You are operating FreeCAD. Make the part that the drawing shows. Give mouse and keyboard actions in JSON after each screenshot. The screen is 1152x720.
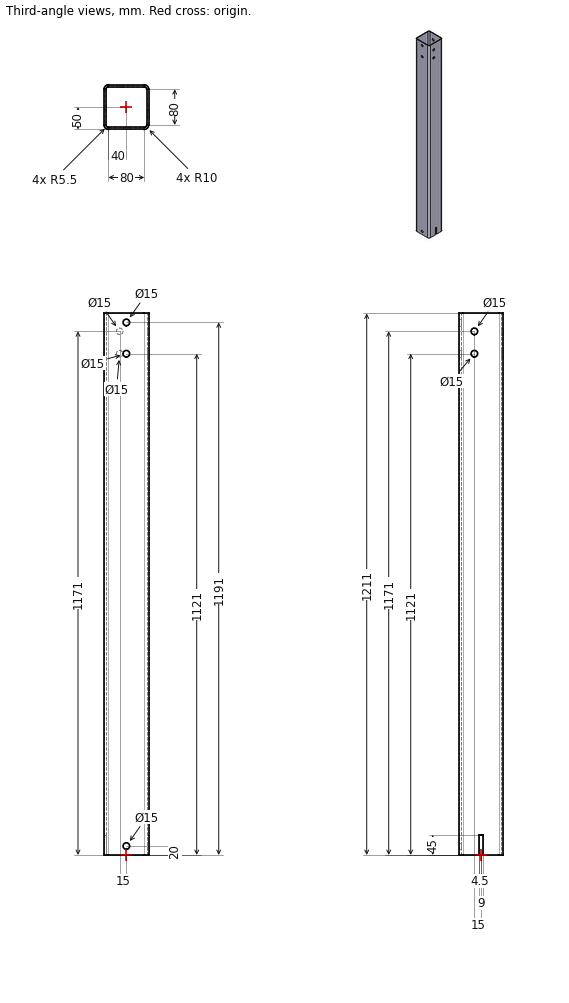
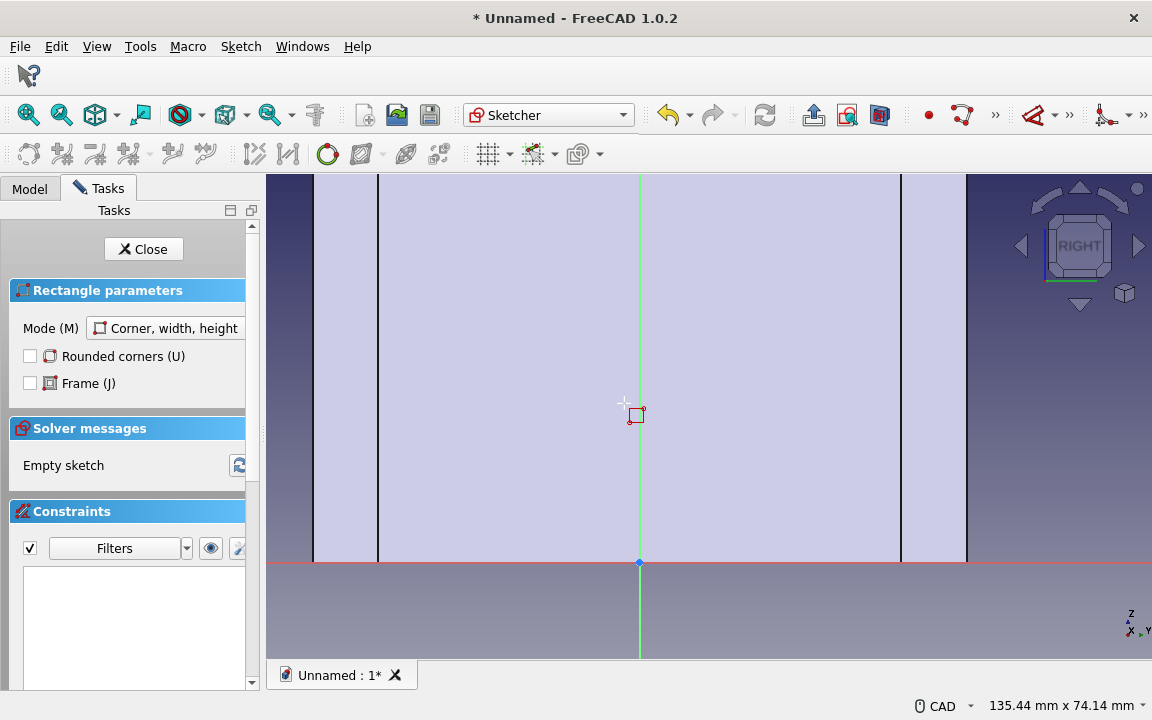
{"action": "left_click", "coordinate": [610, 268]}
{"action": "left_click", "coordinate": [669, 563]}
{"action": "key", "text": "Escape"}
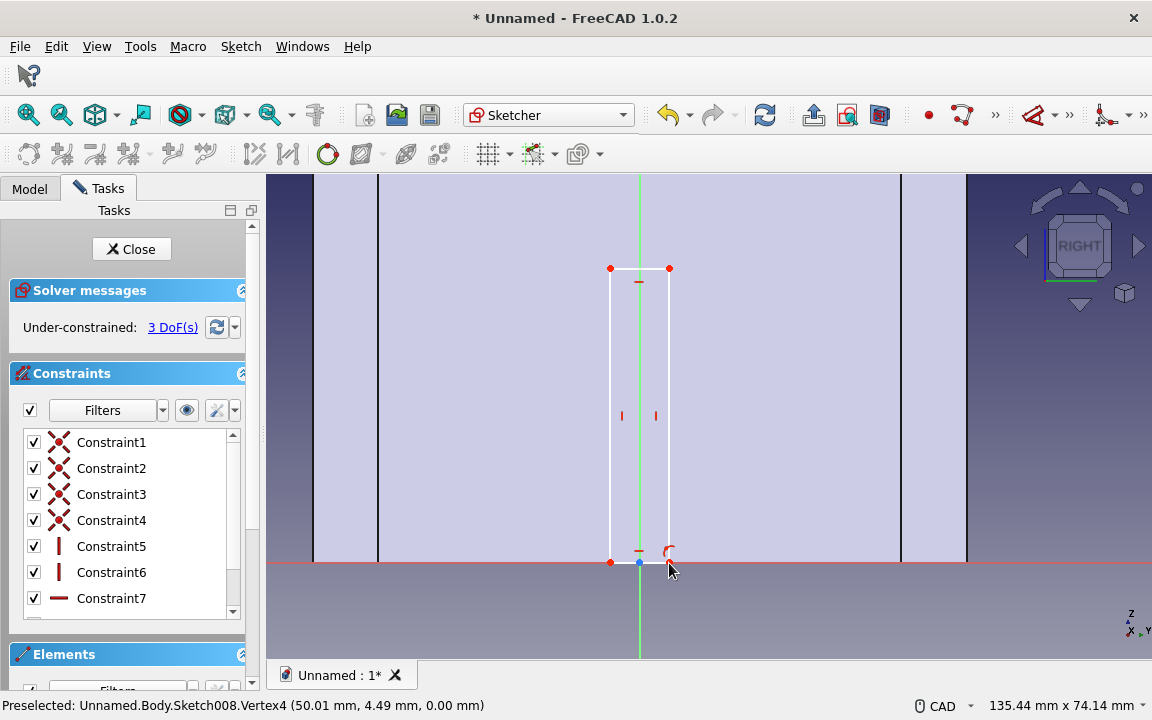
{"action": "key", "text": "d"}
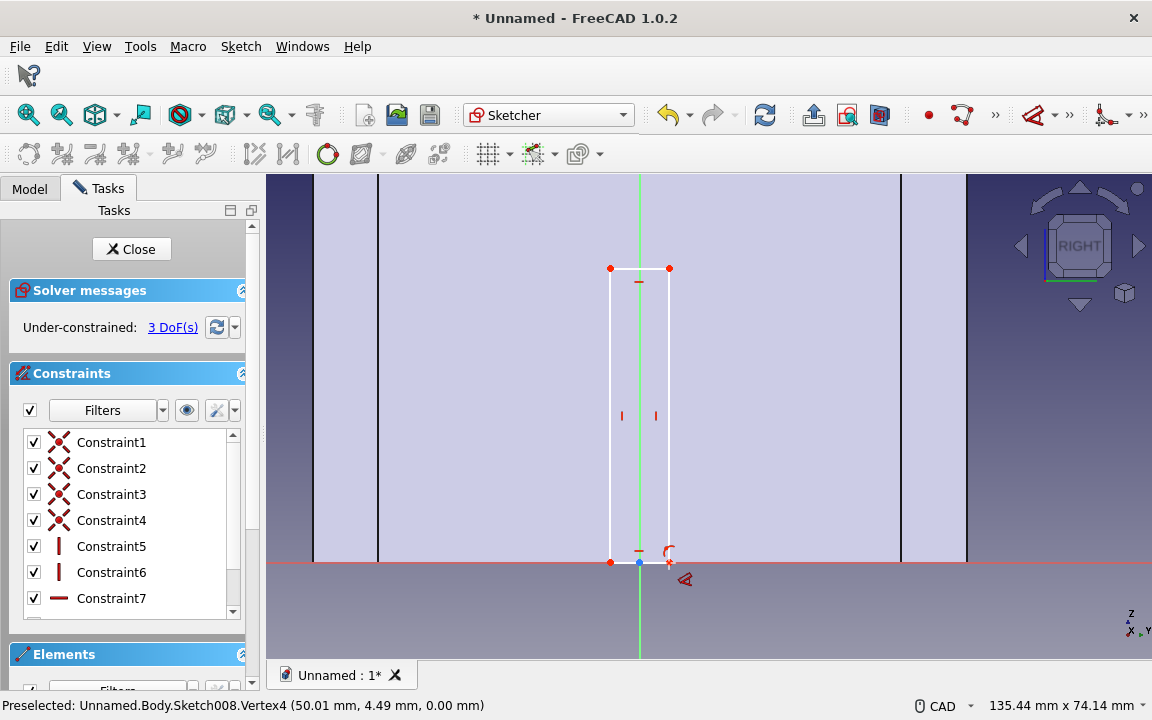
{"action": "left_click", "coordinate": [628, 563]}
{"action": "left_click", "coordinate": [626, 597]}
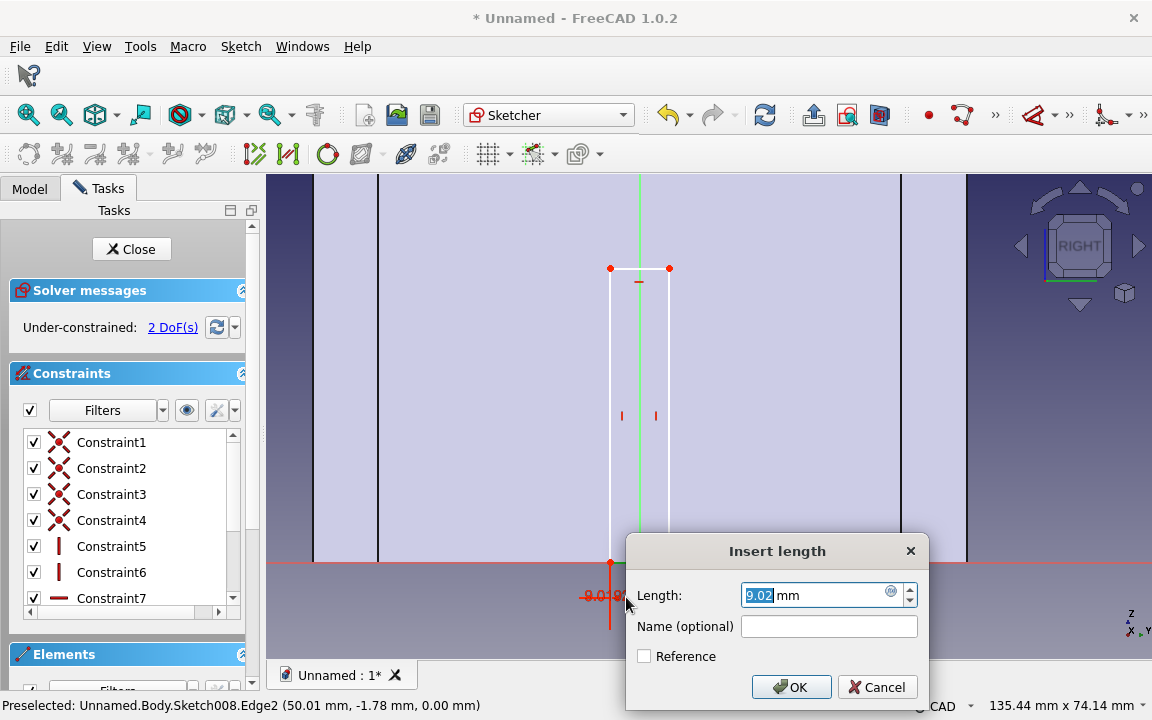
{"action": "type", "text": "9"}
{"action": "key", "text": "Return"}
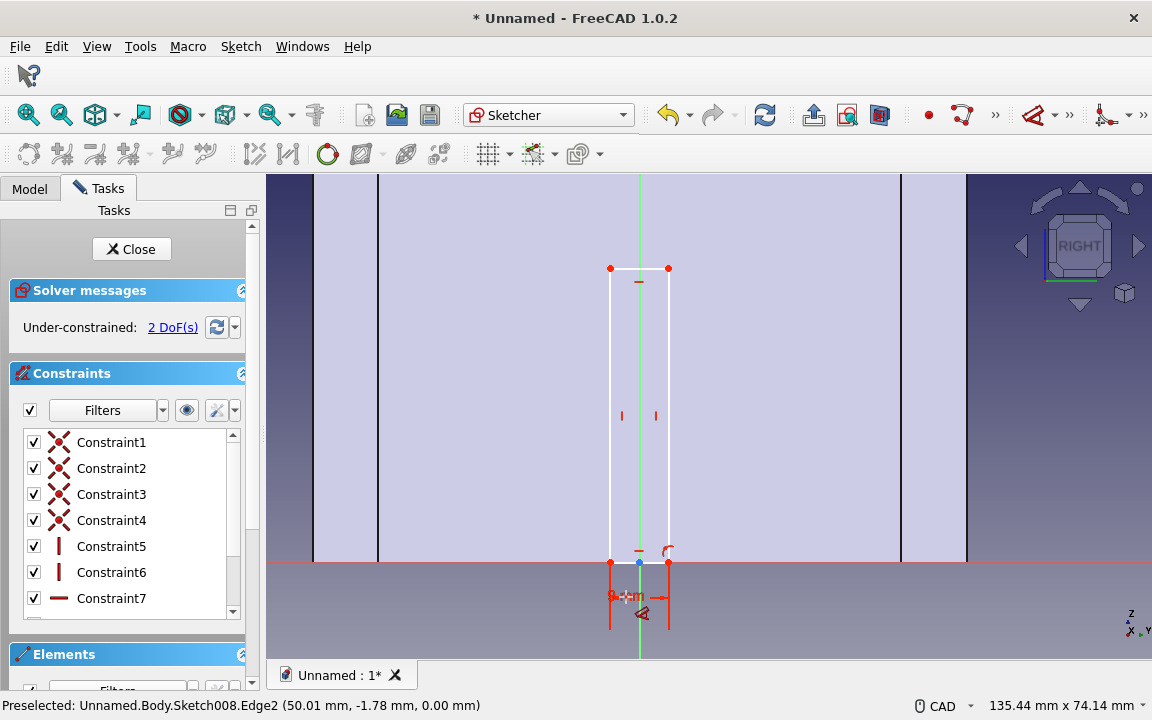
{"action": "left_click", "coordinate": [610, 357]}
{"action": "left_click", "coordinate": [576, 416]}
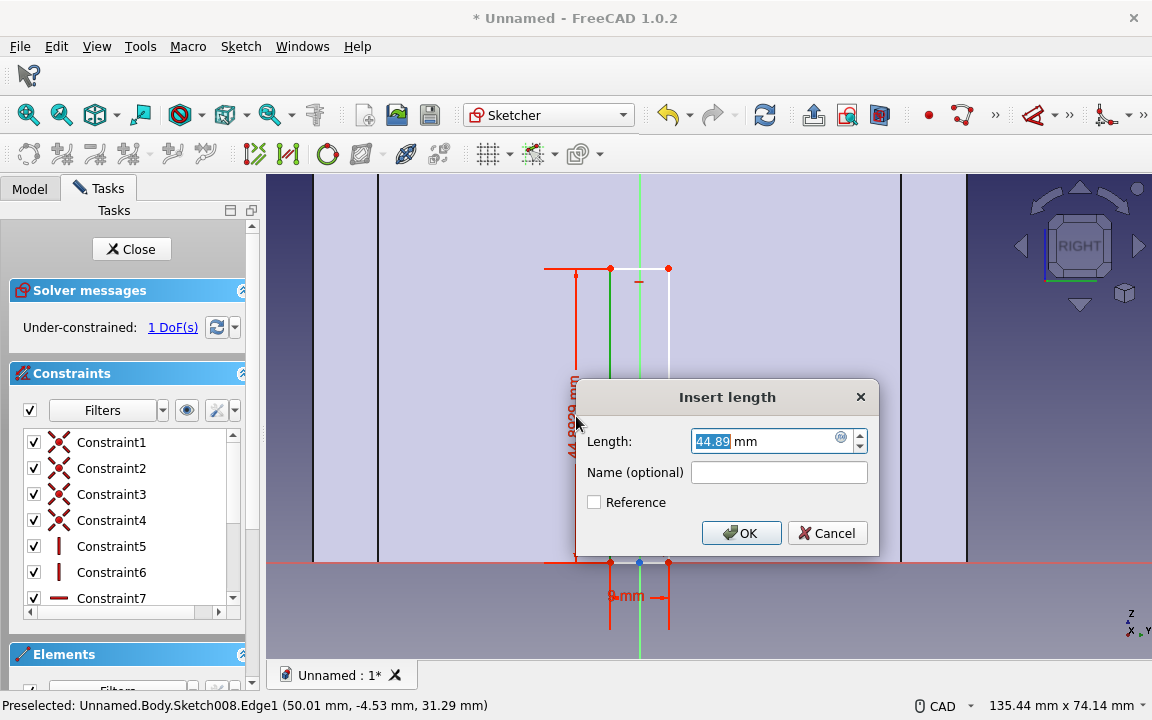
{"action": "type", "text": "45"}
{"action": "key", "text": "Return"}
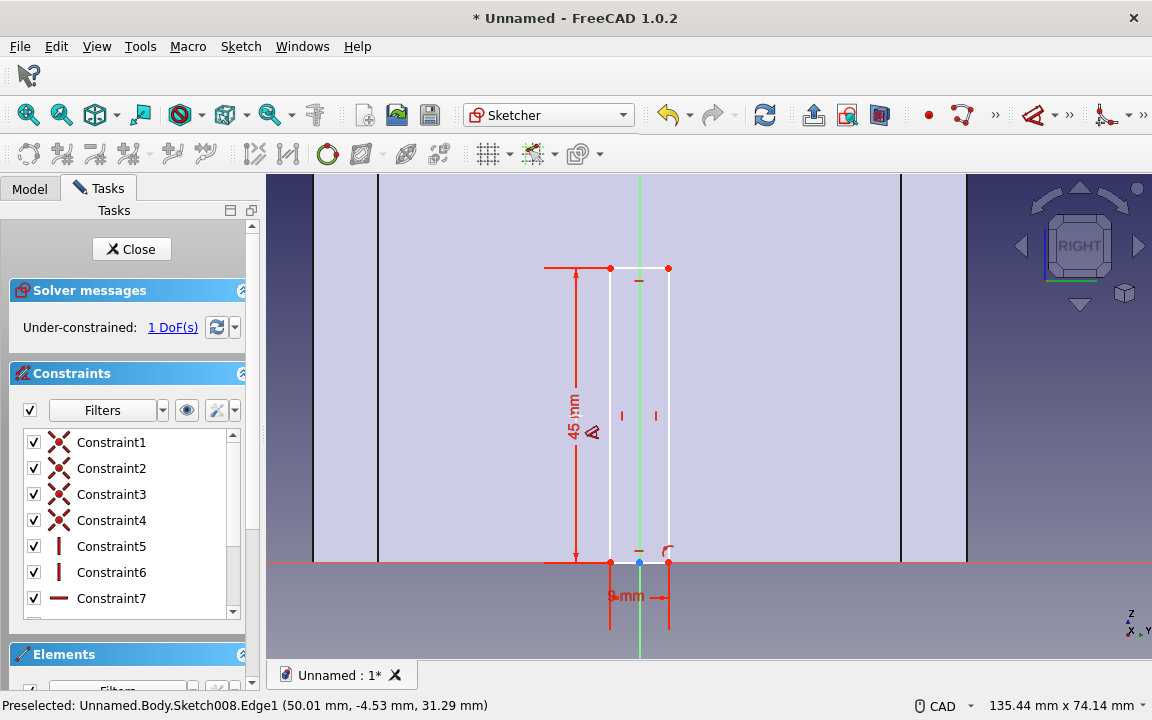
{"action": "scroll", "coordinate": [610, 268], "scroll_direction": "up", "scroll_amount": 2}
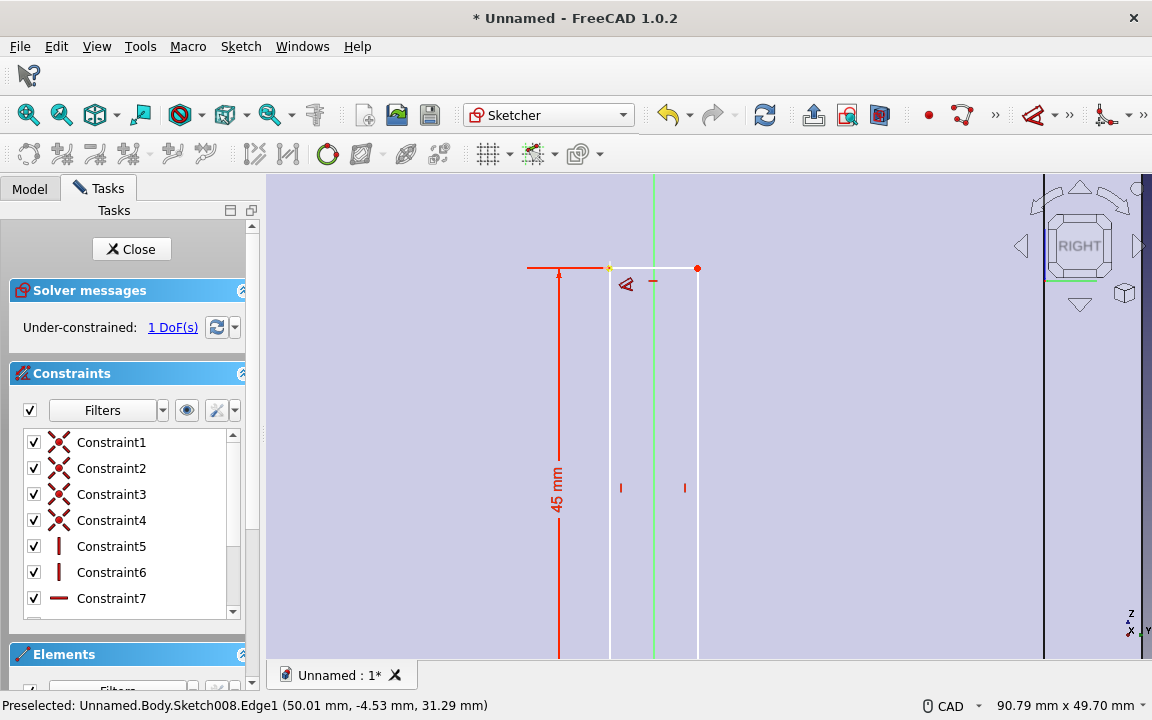
{"action": "left_click", "coordinate": [610, 268]}
{"action": "left_click", "coordinate": [632, 234]}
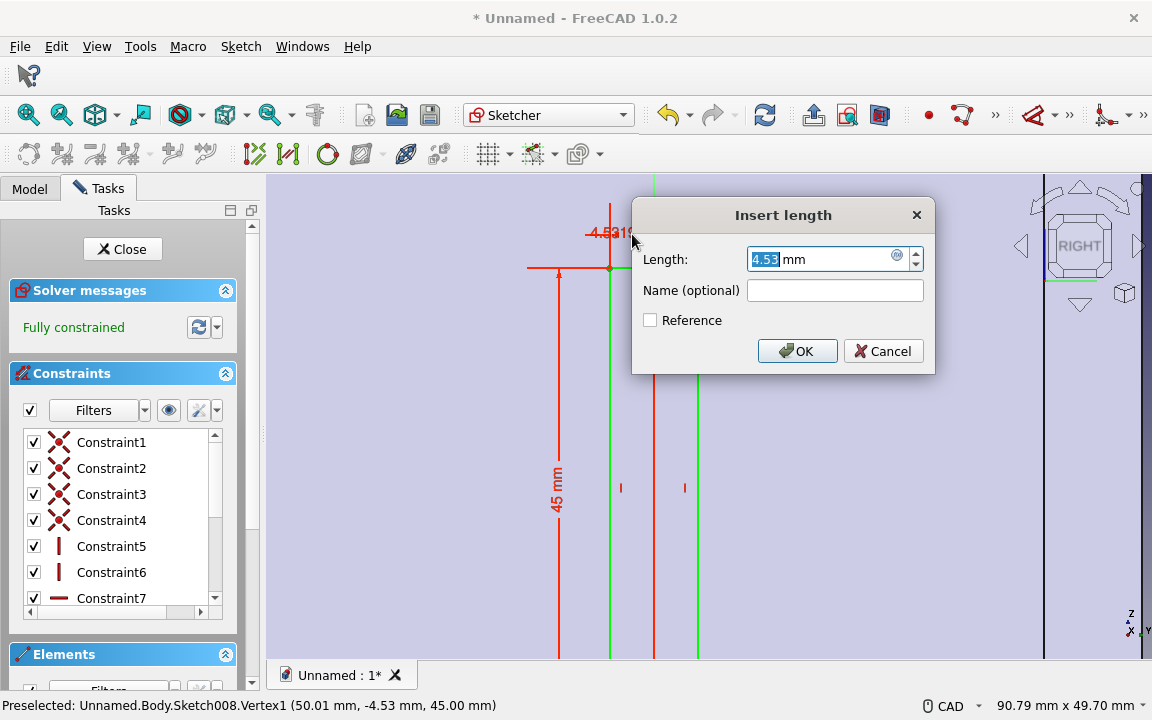
{"action": "type", "text": "4.5"}
{"action": "key", "text": "Return"}
{"action": "key", "text": "Escape"}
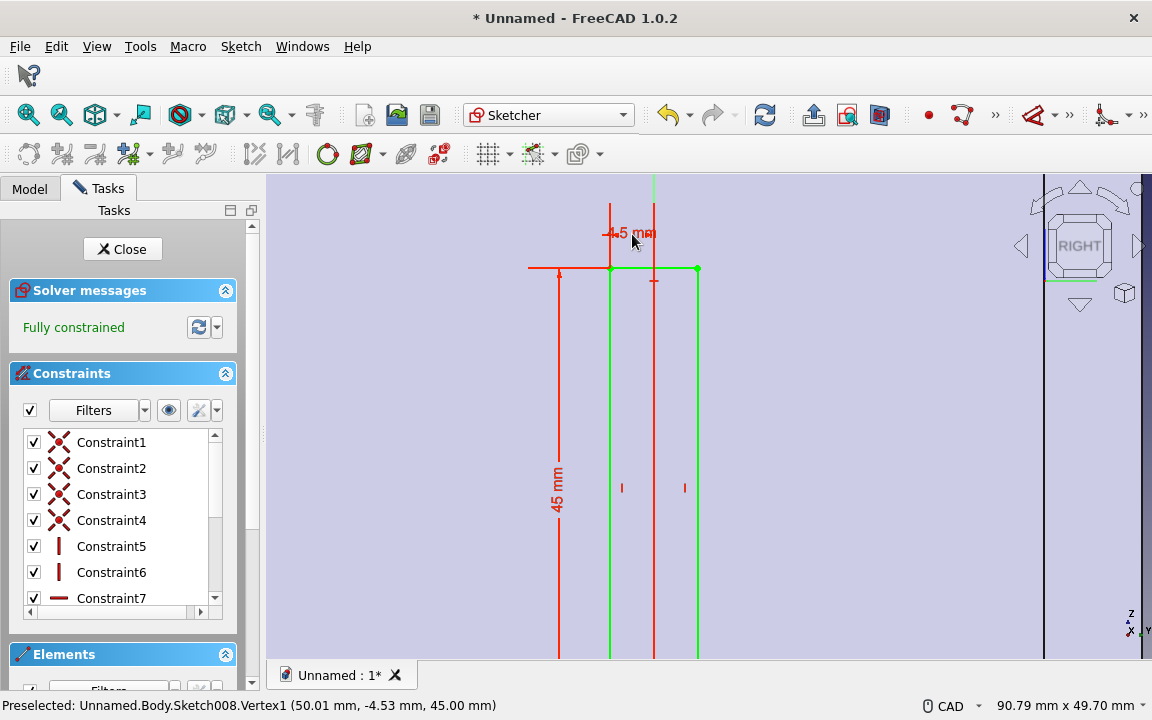
{"action": "left_click", "coordinate": [123, 249]}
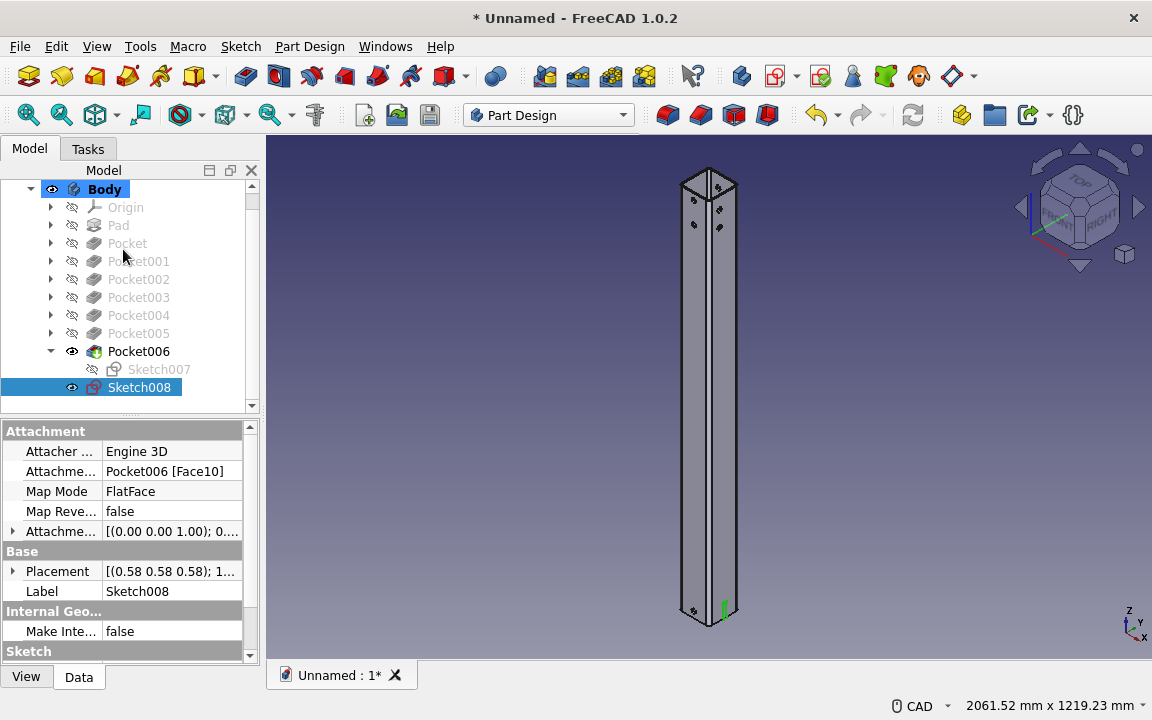
{"action": "left_click", "coordinate": [246, 76]}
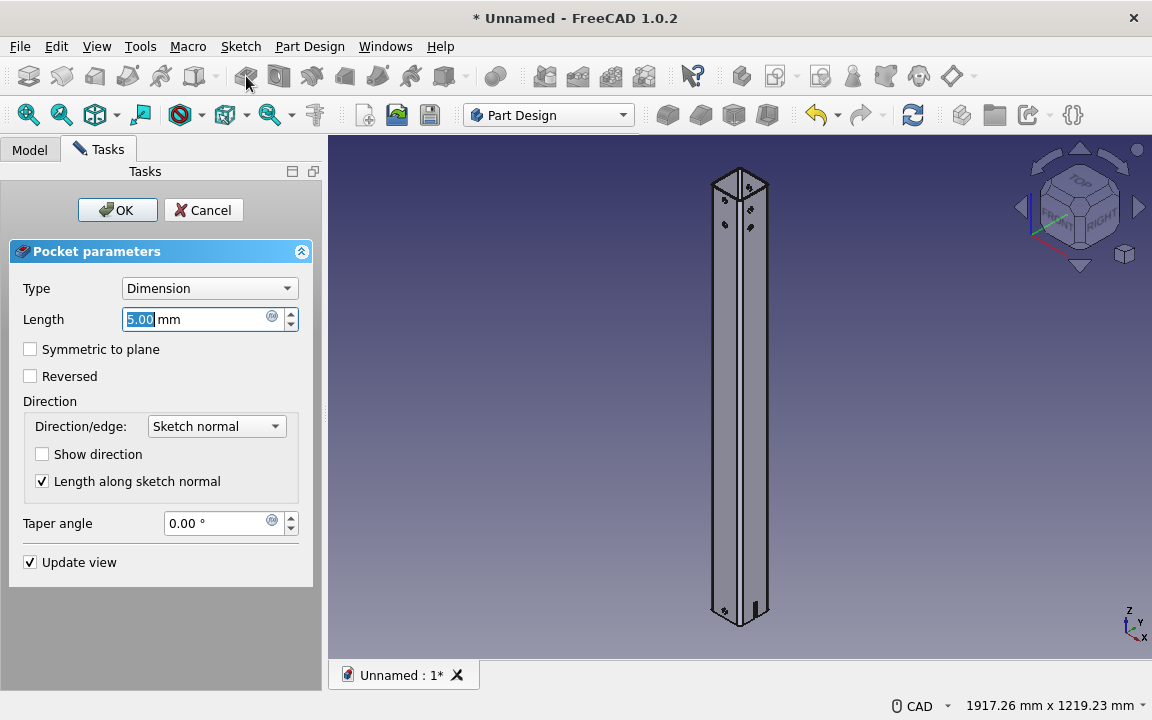
{"action": "left_click", "coordinate": [210, 288]}